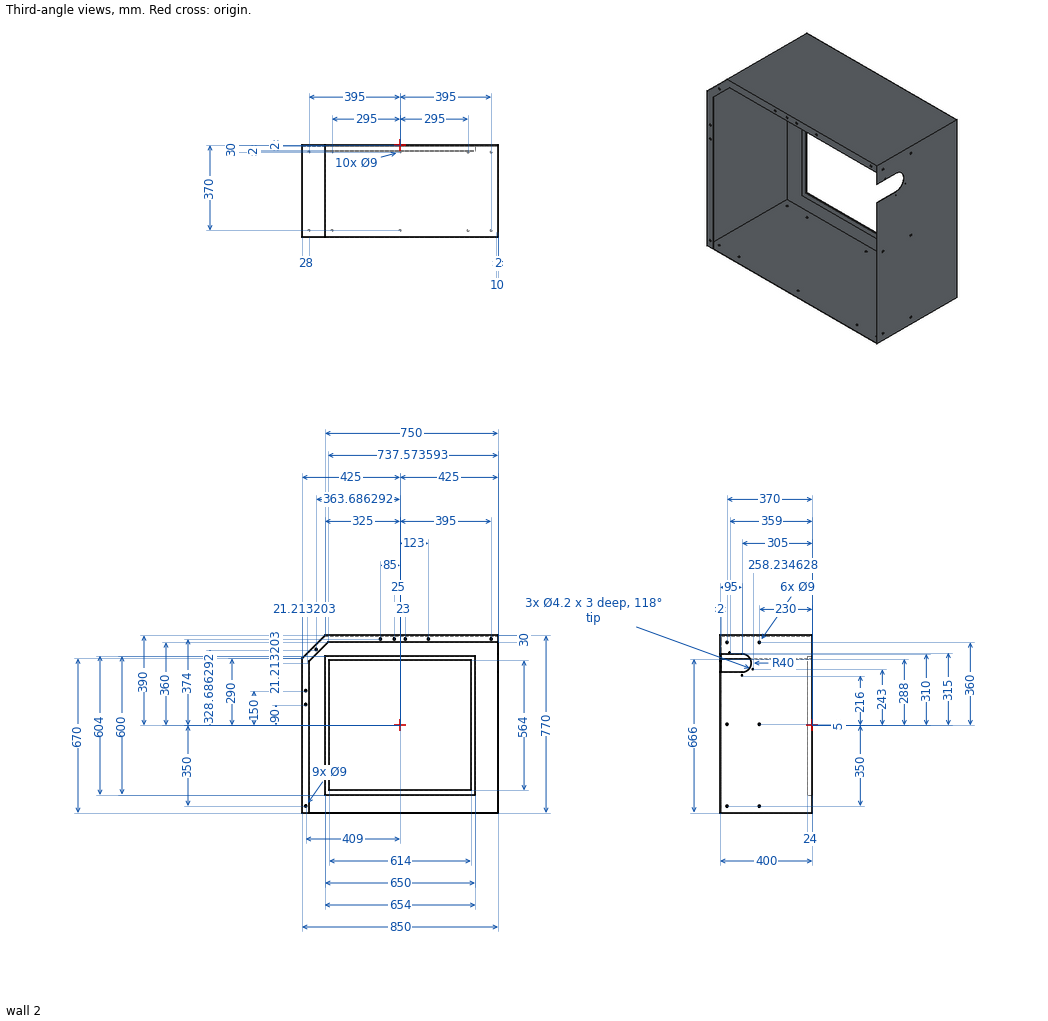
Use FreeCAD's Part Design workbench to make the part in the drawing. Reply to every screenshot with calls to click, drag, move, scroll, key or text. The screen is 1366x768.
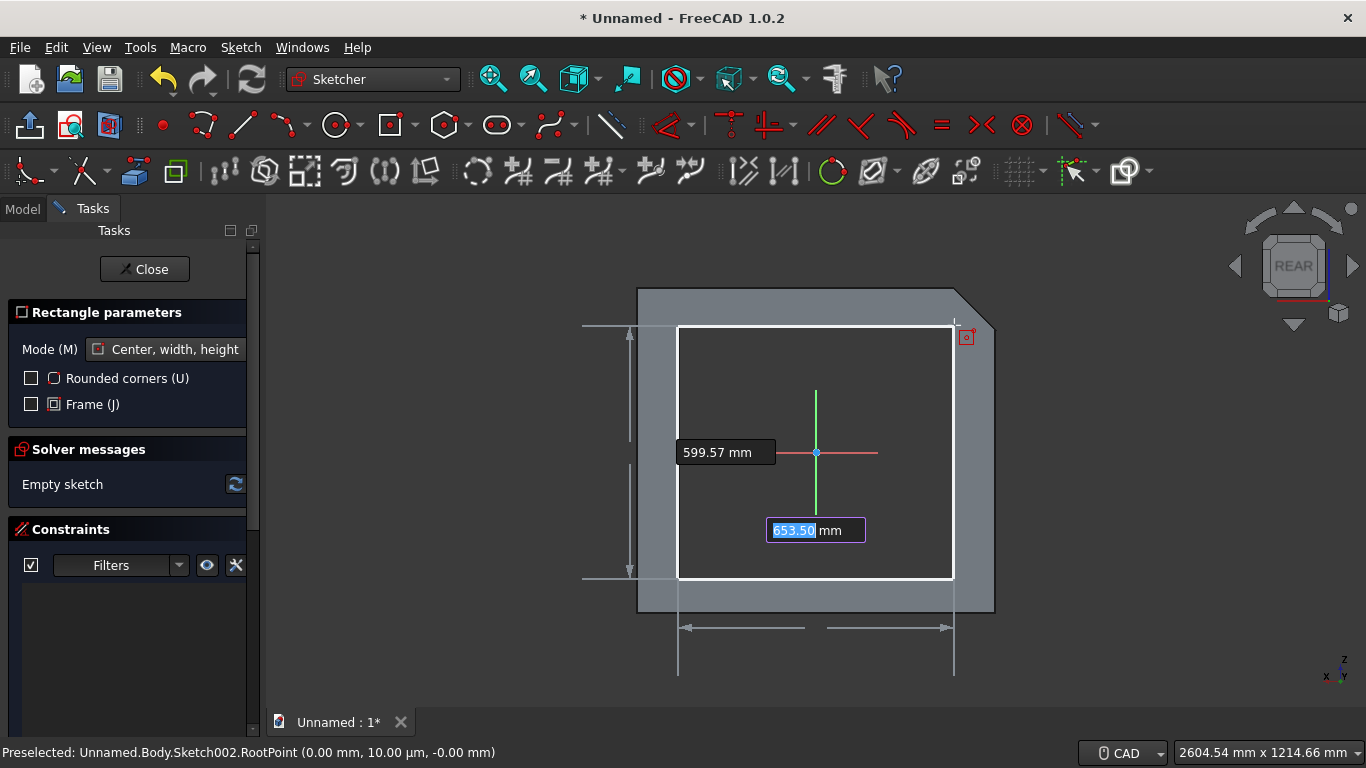
text(654)
key(Tab)
text(604)
key(Return)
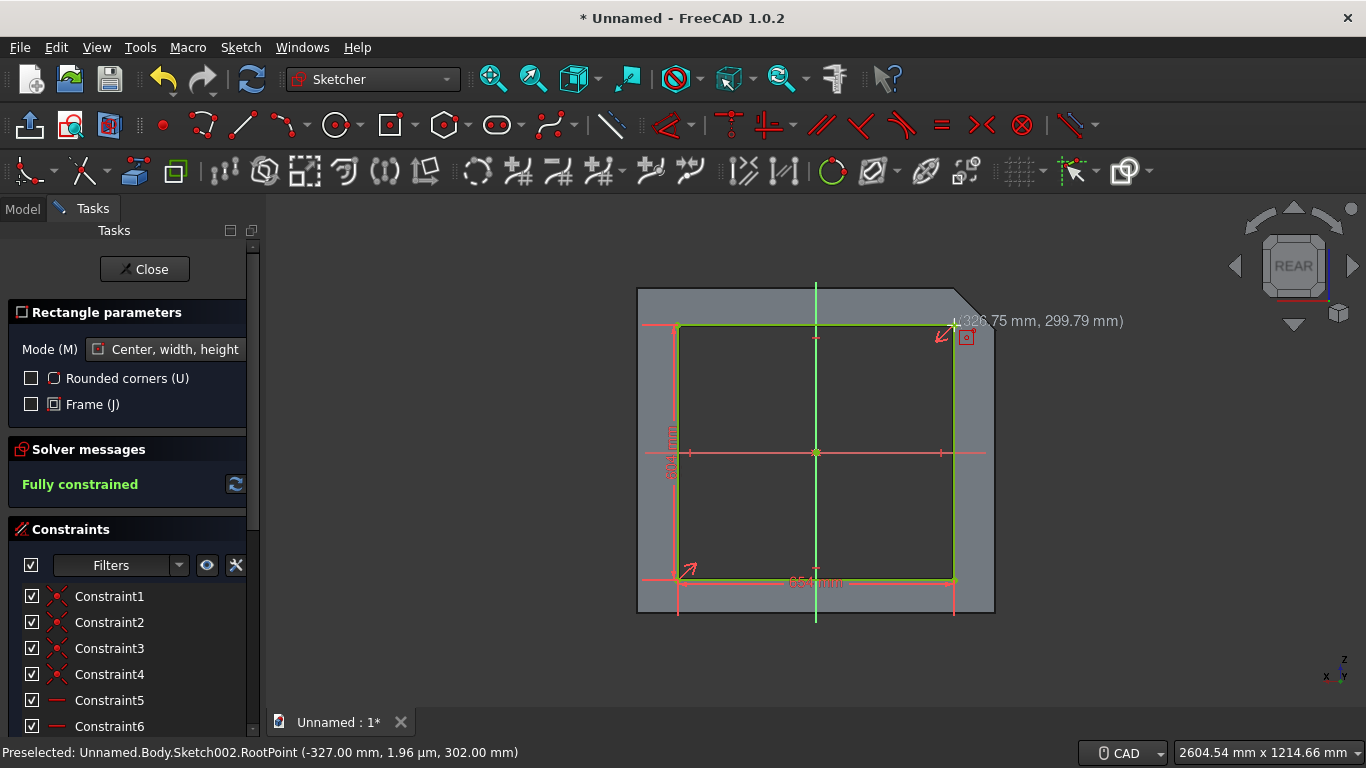
click(816, 453)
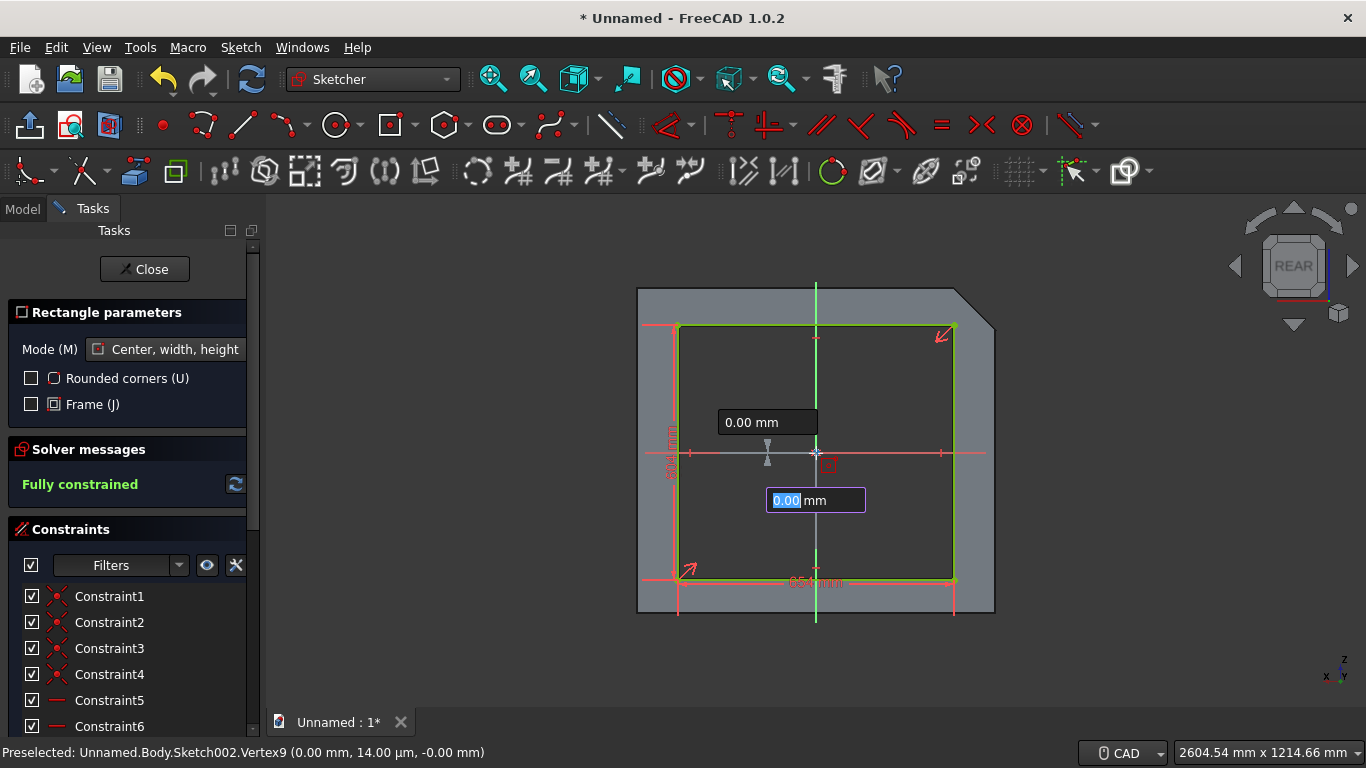
scroll(953, 326, up, 15)
move(946, 319)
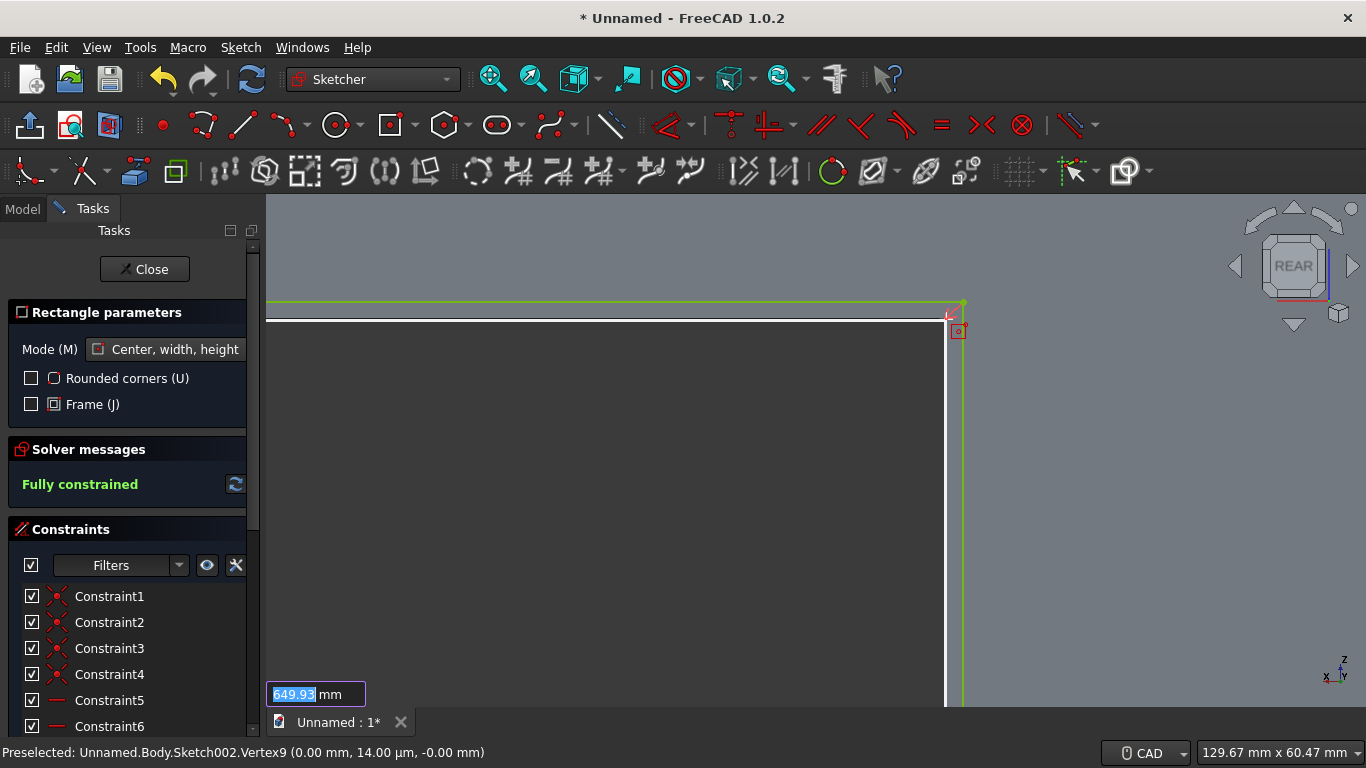
text(650)
key(Tab)
text(600)
key(Return)
key(Escape)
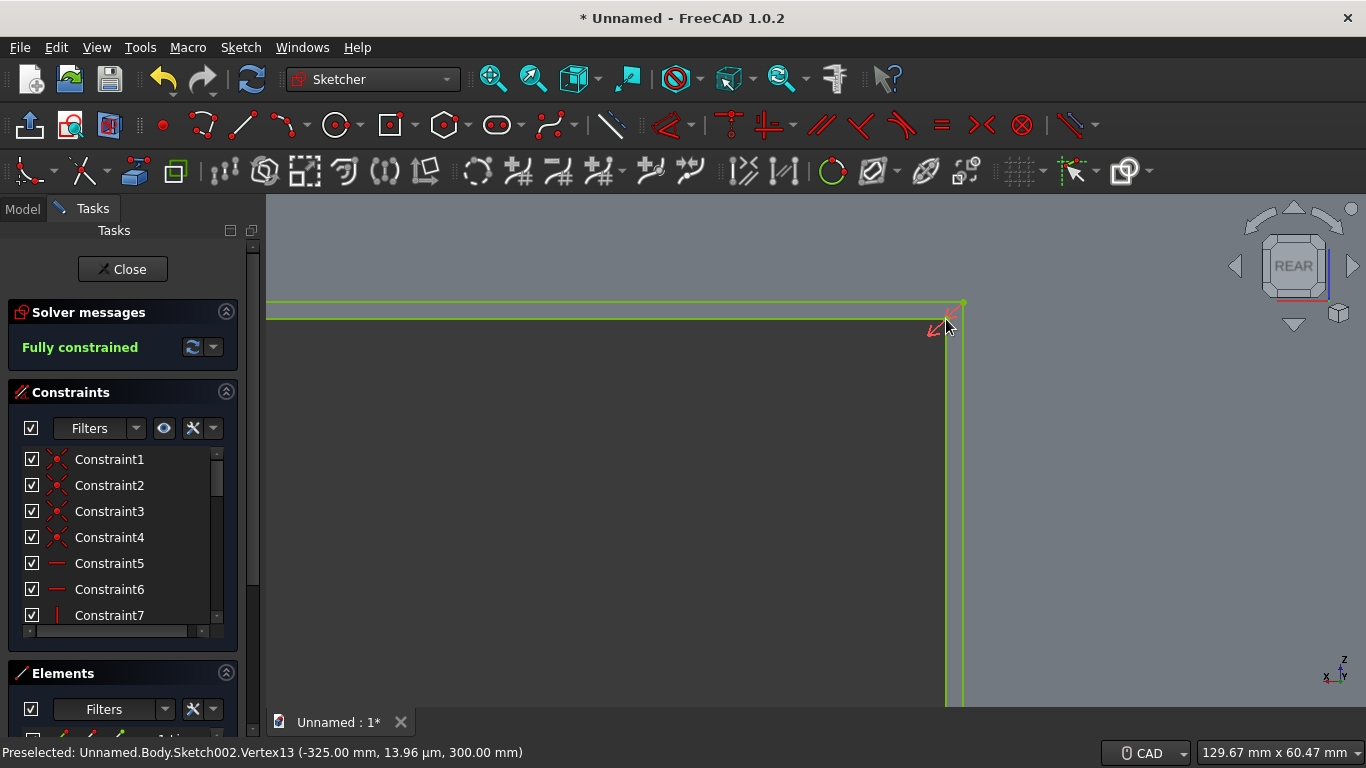
click(123, 269)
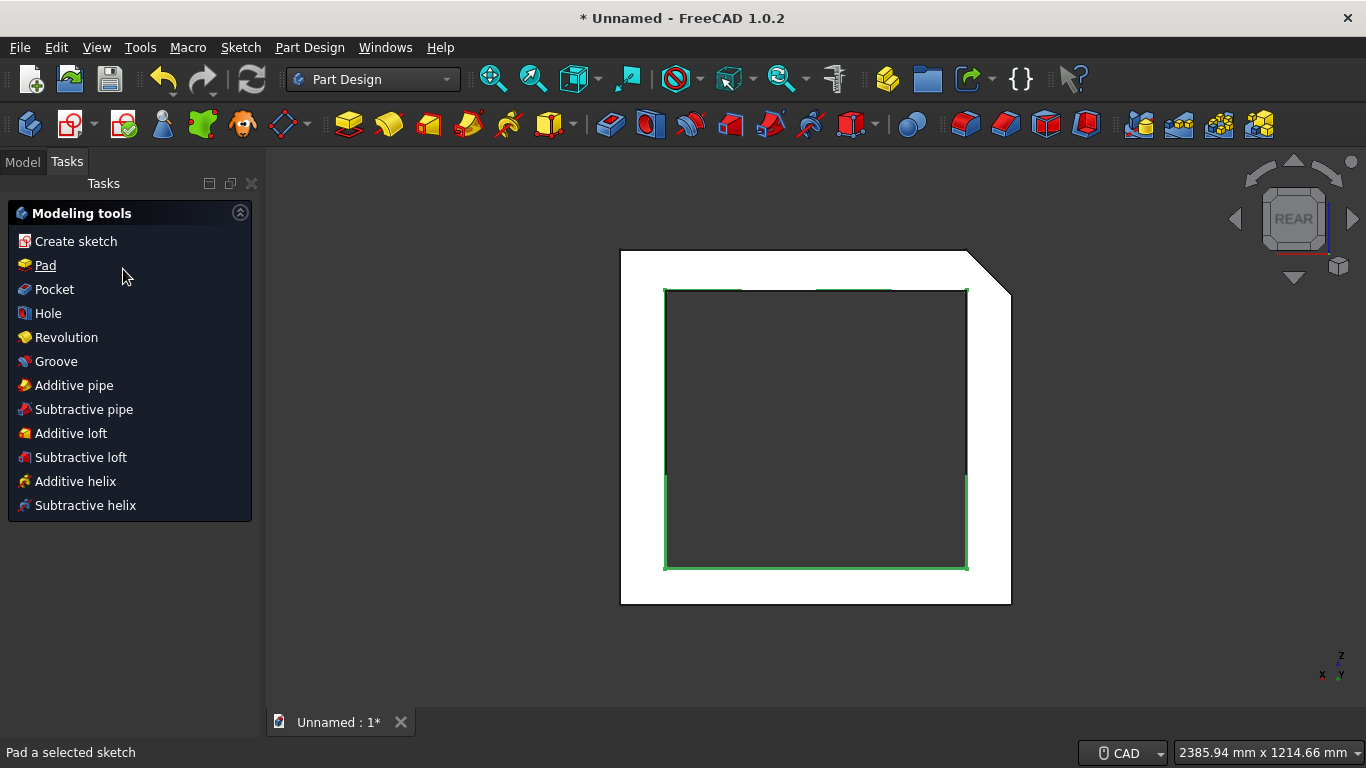
click(350, 124)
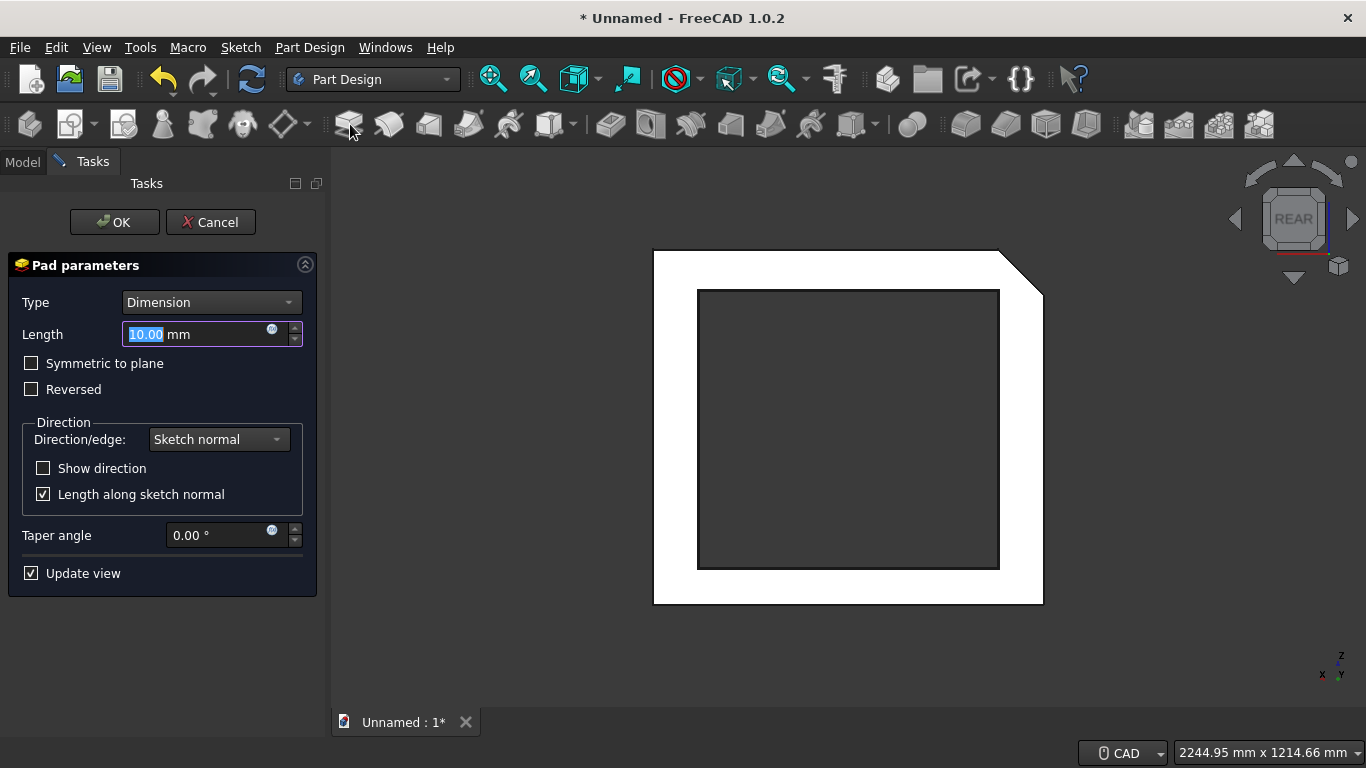
text(24)
key(Tab)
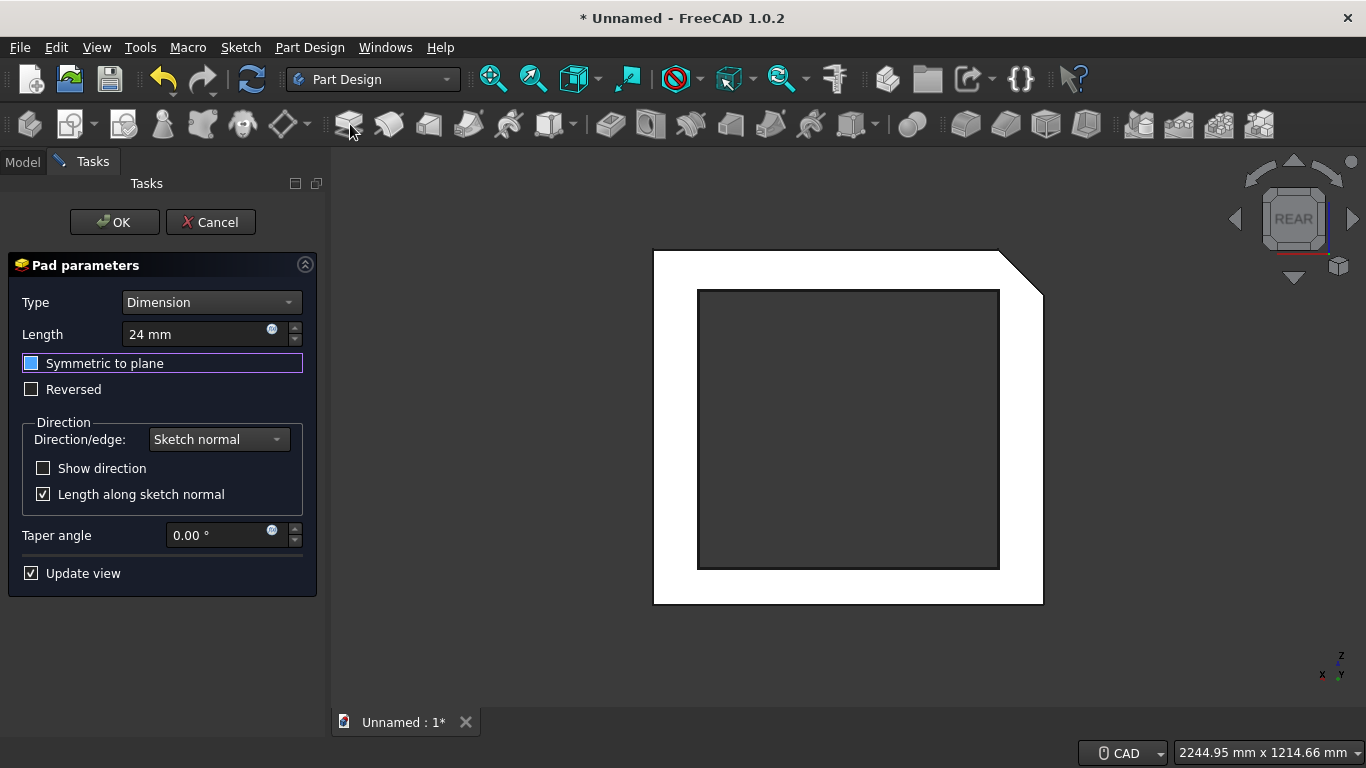
click(30, 389)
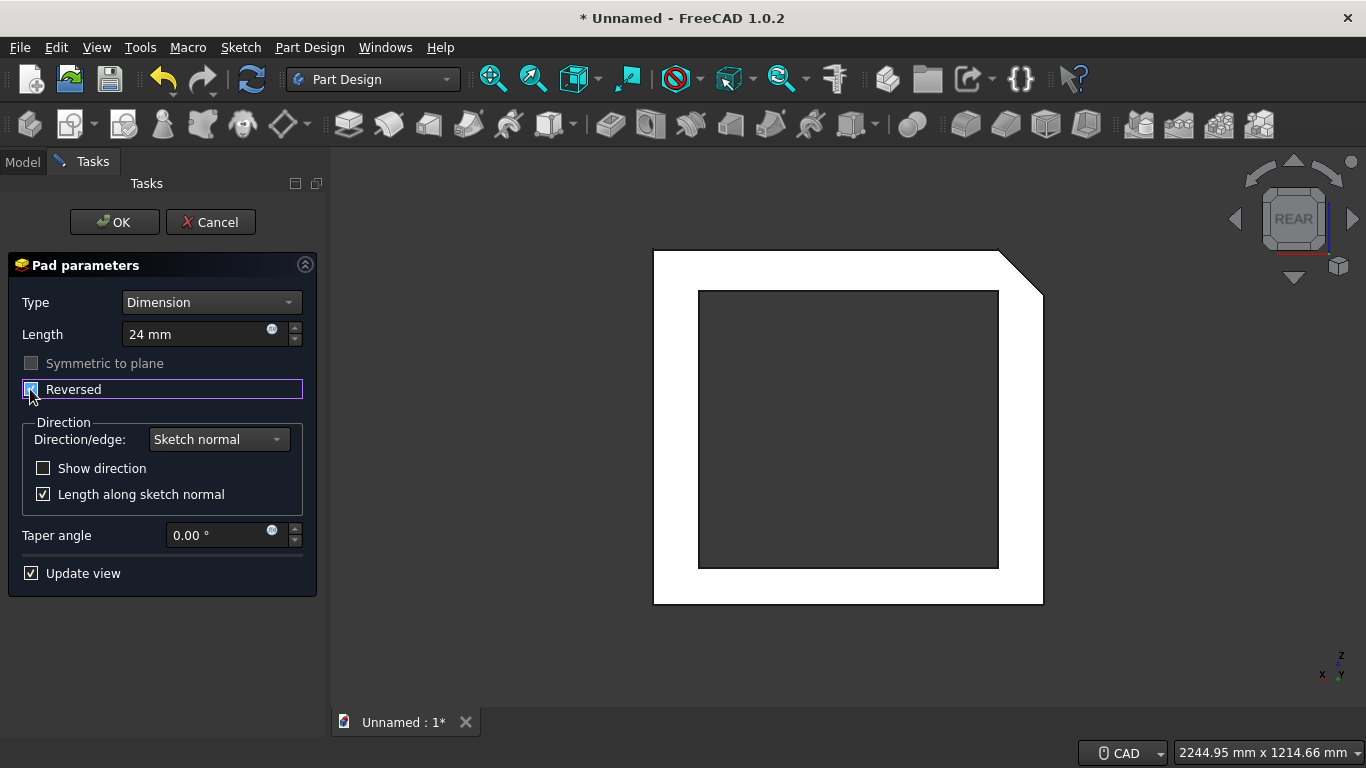
click(115, 222)